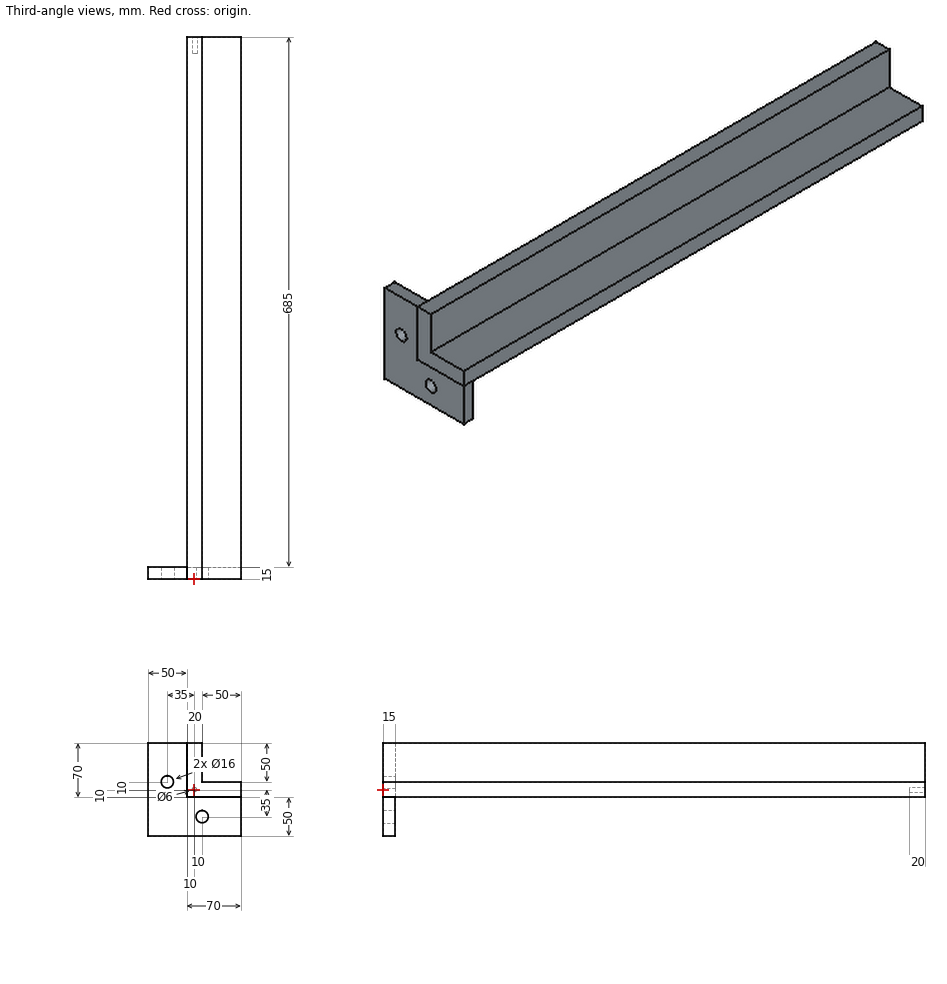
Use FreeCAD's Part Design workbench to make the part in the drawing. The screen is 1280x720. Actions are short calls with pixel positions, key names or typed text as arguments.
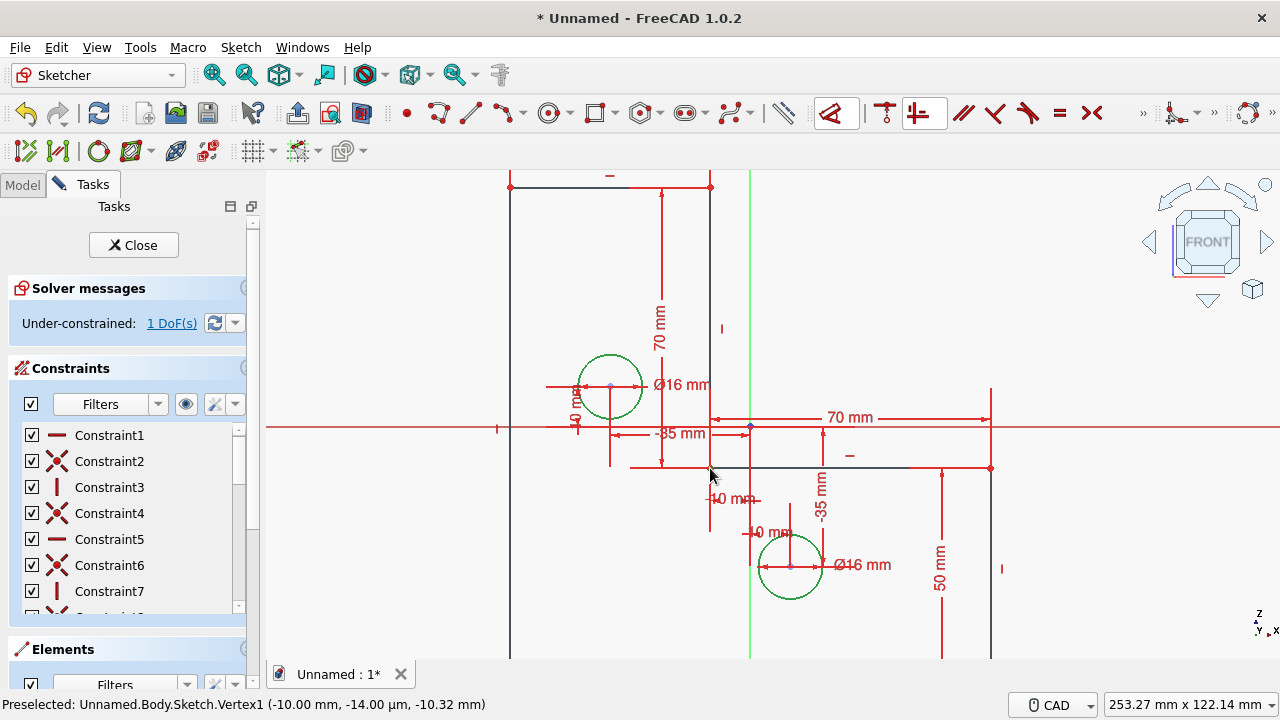
click(854, 114)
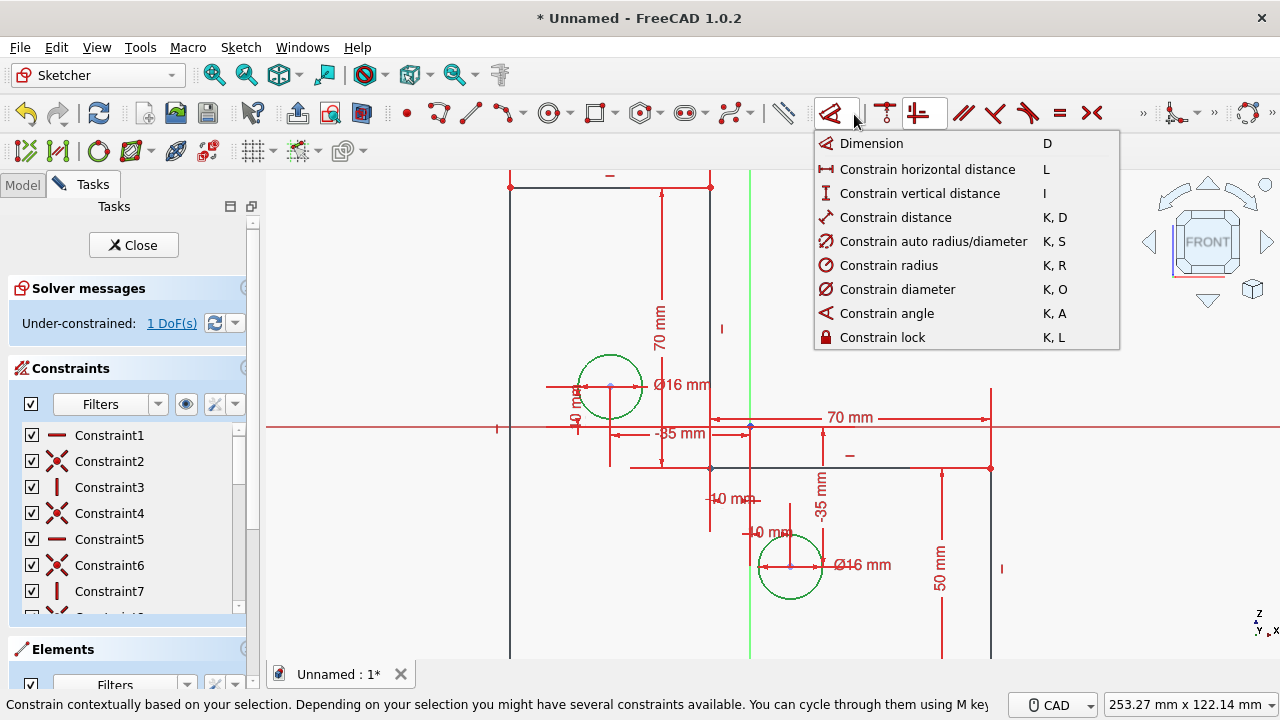
click(967, 193)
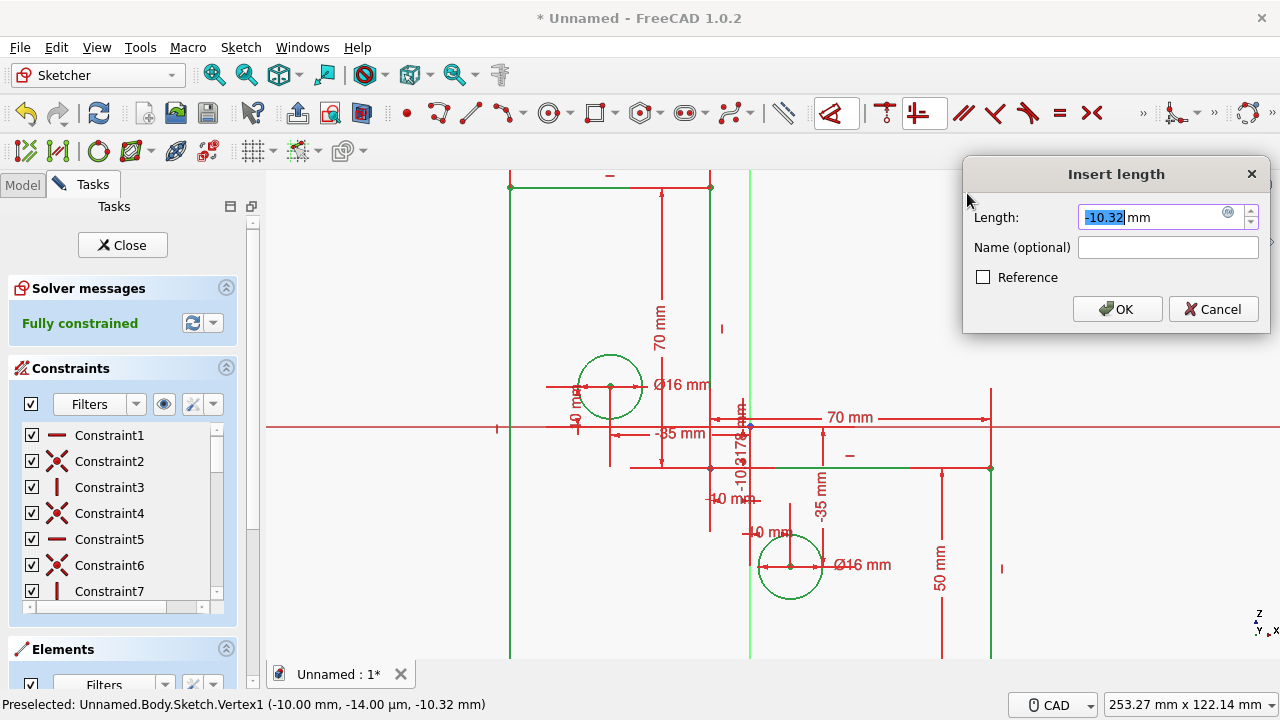
text(-10)
key(Return)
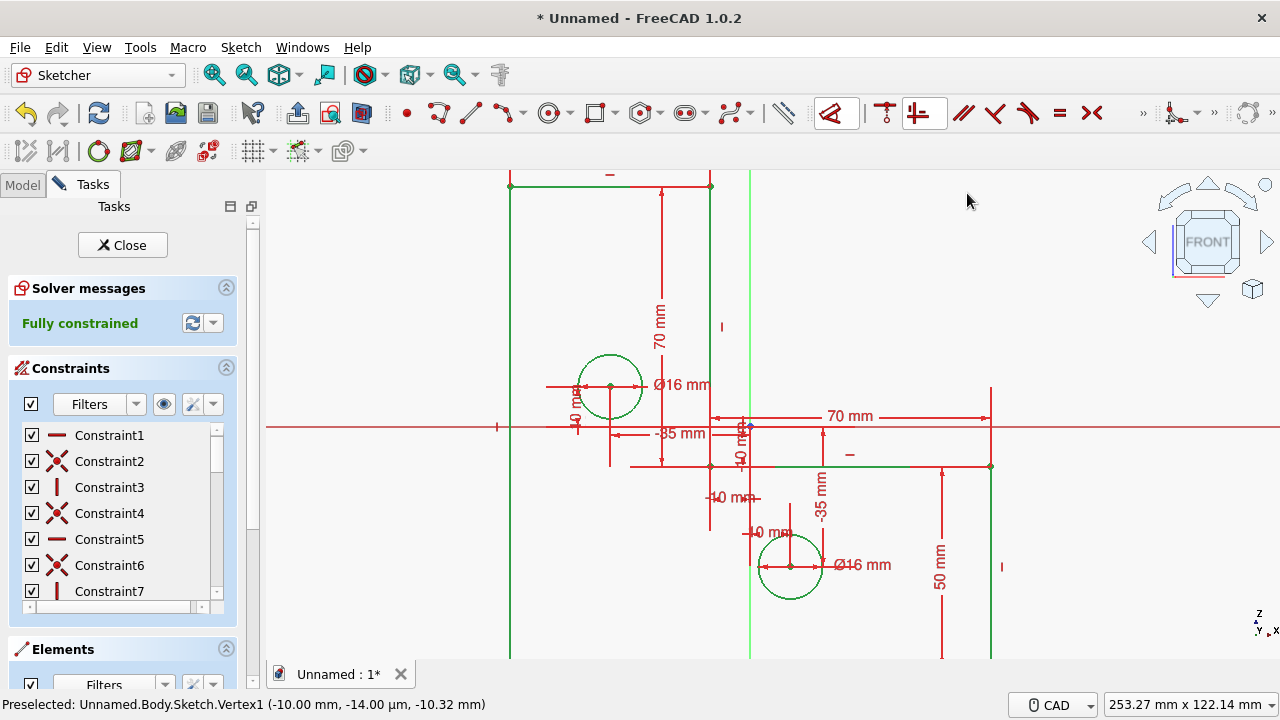
click(123, 245)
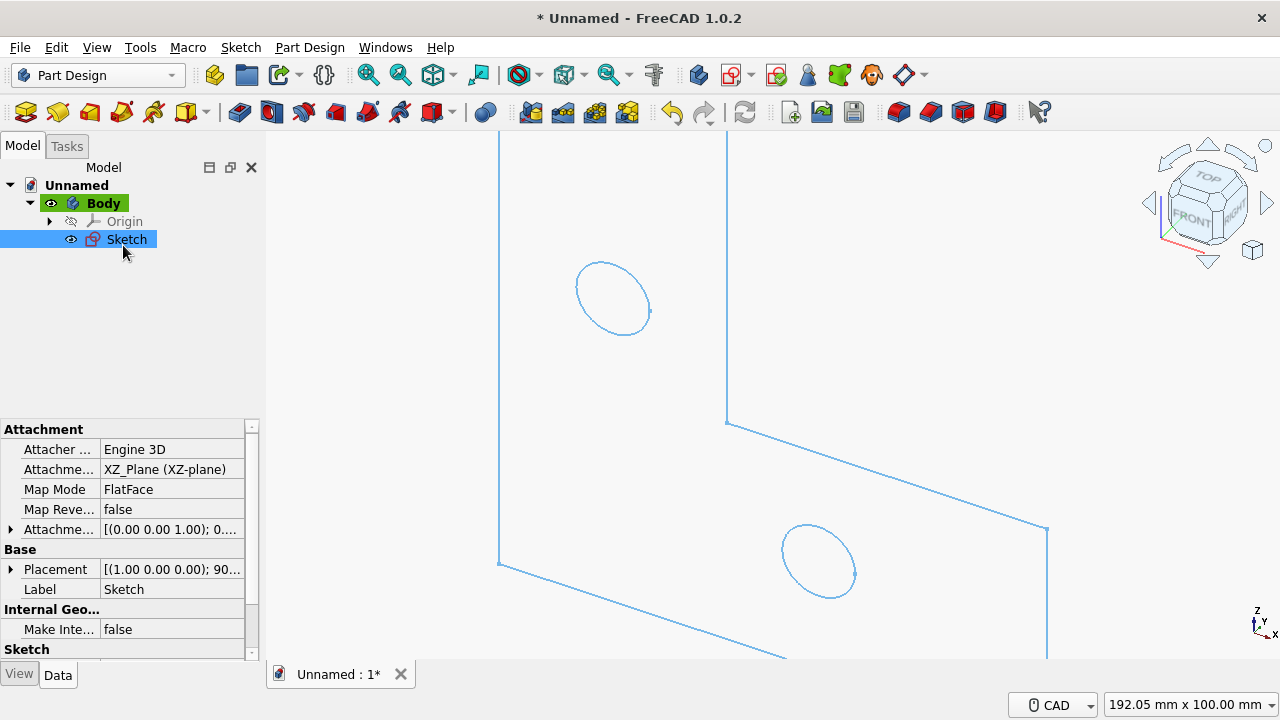
click(26, 112)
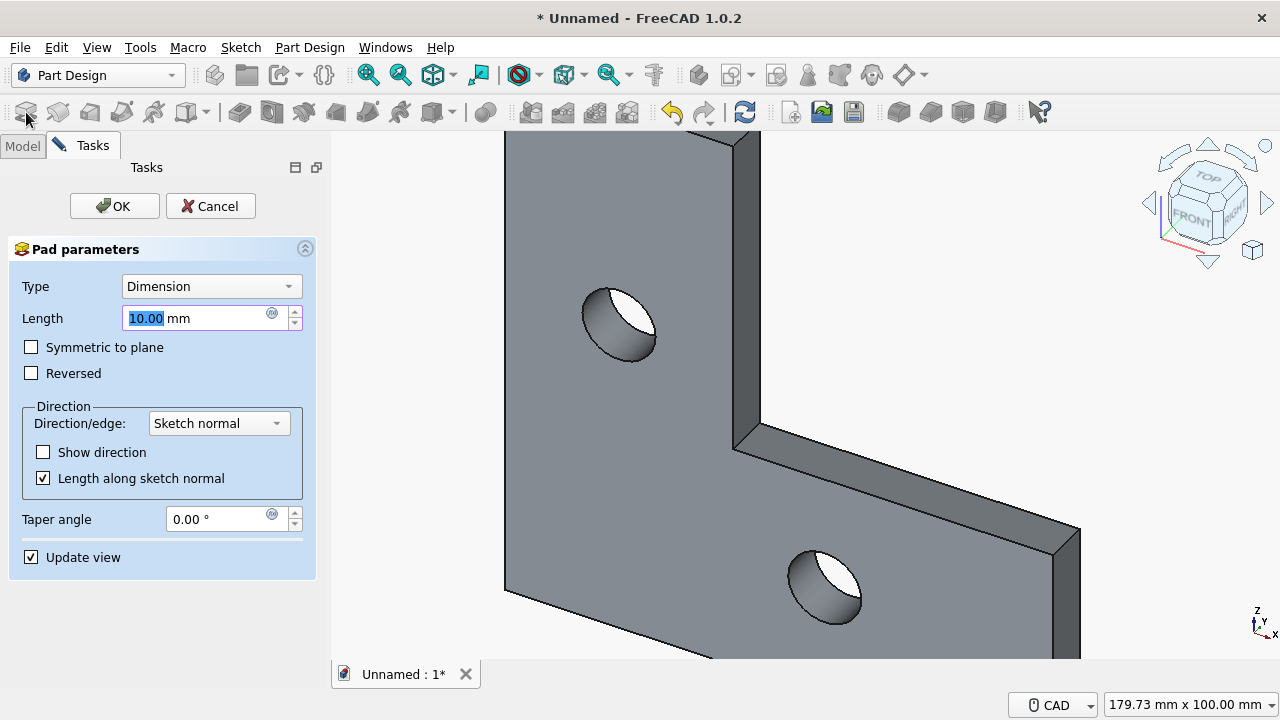
text(15)
key(Tab)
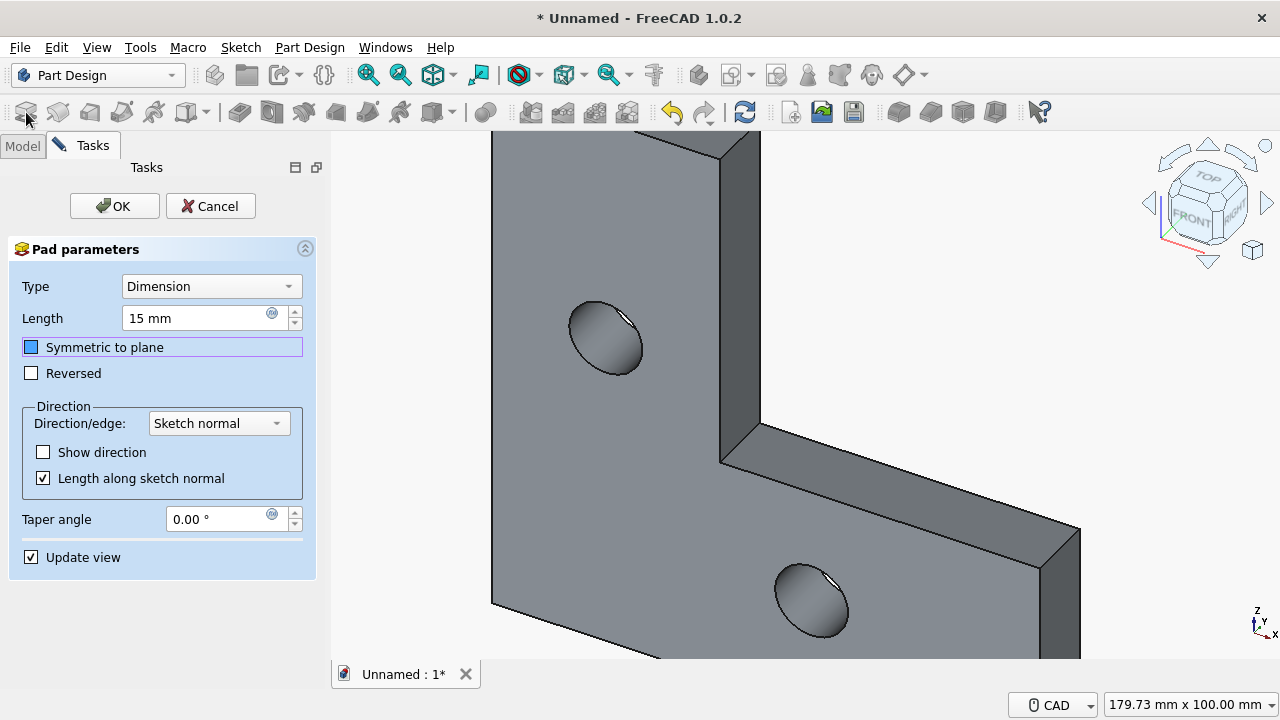
click(30, 373)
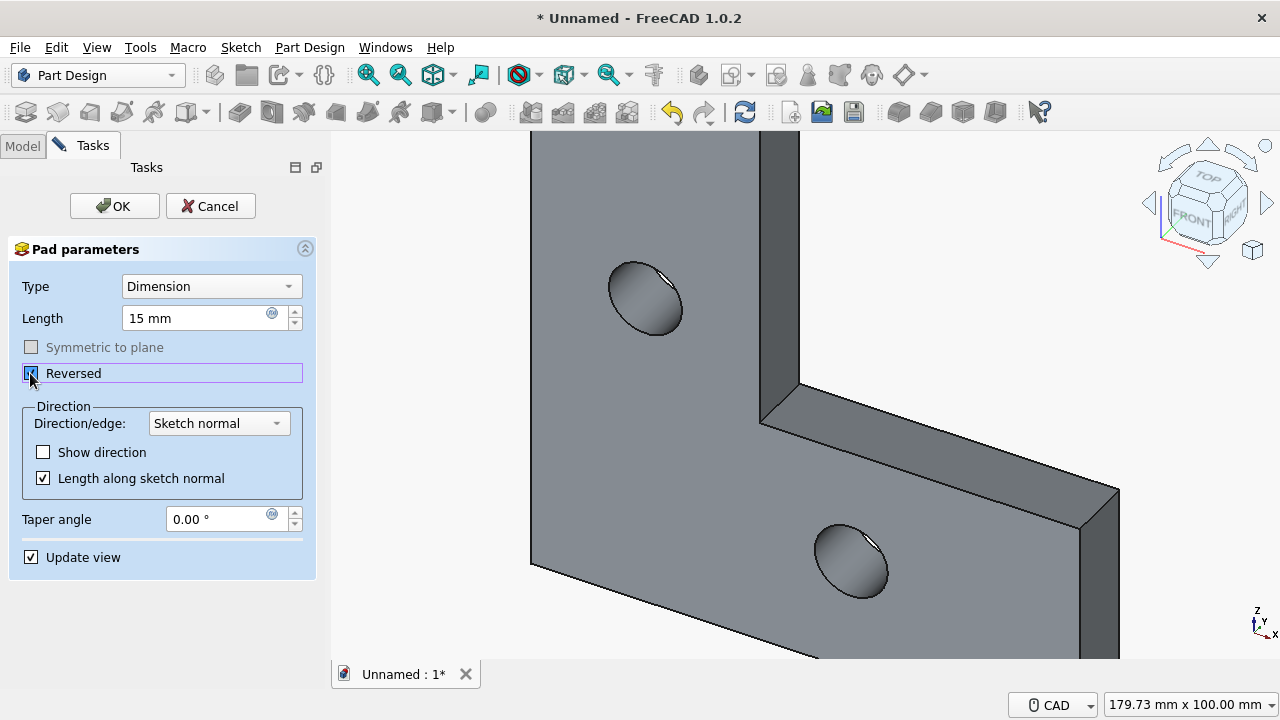
click(115, 206)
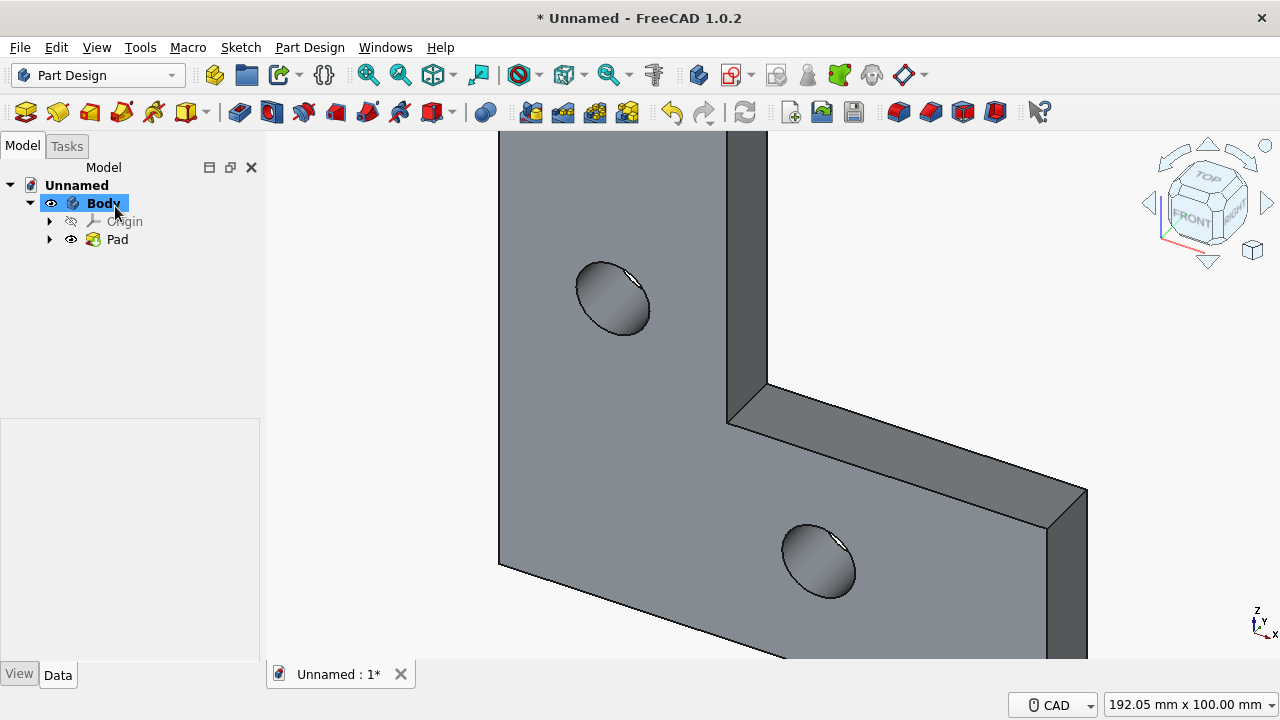
click(370, 76)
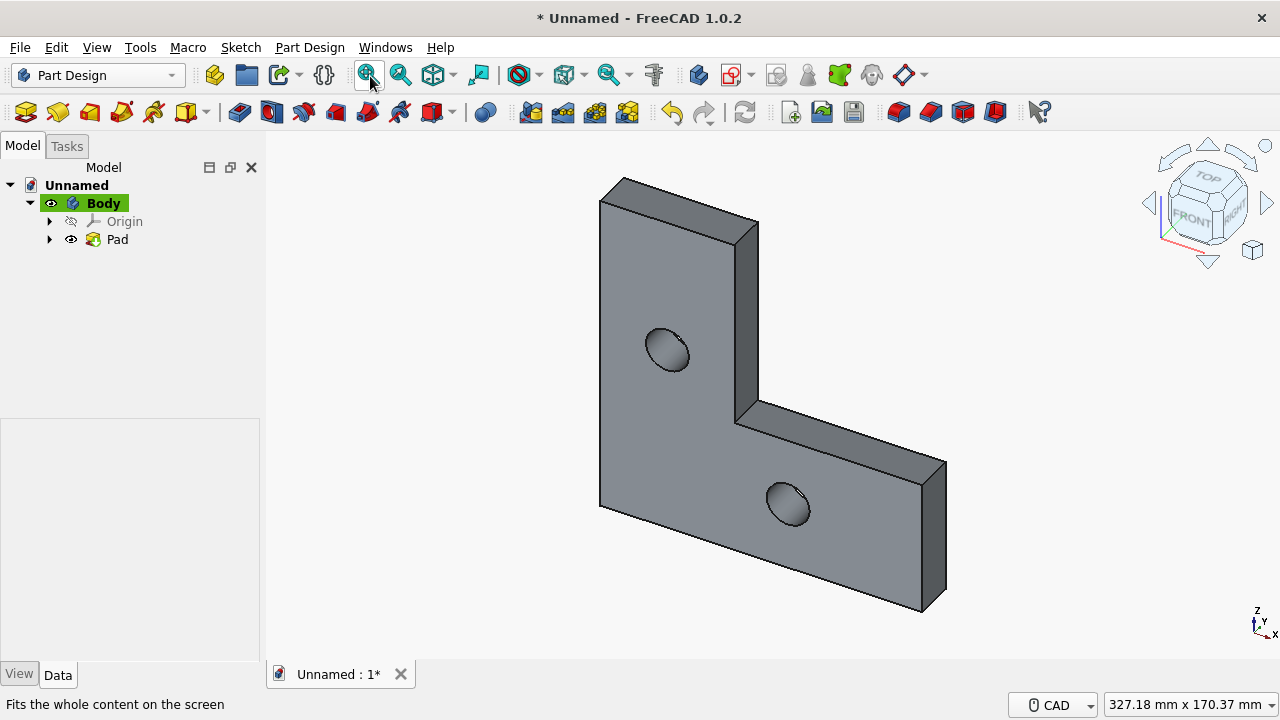
click(700, 76)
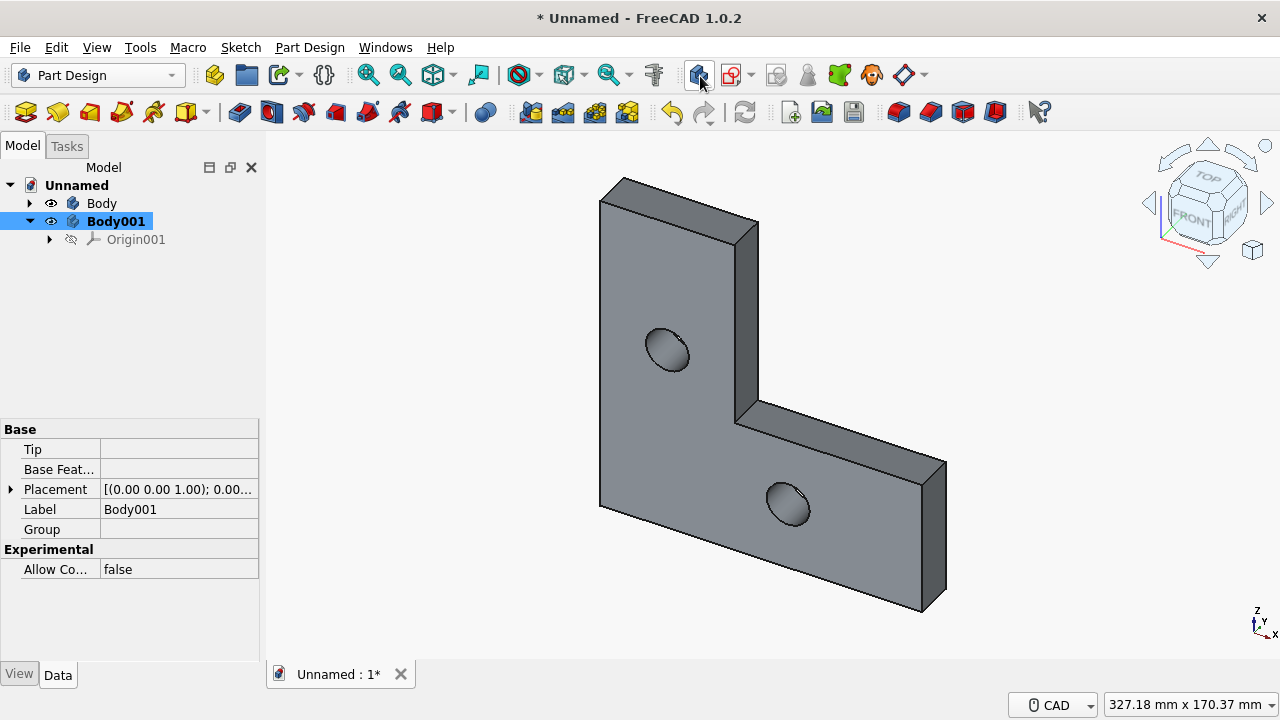
click(50, 239)